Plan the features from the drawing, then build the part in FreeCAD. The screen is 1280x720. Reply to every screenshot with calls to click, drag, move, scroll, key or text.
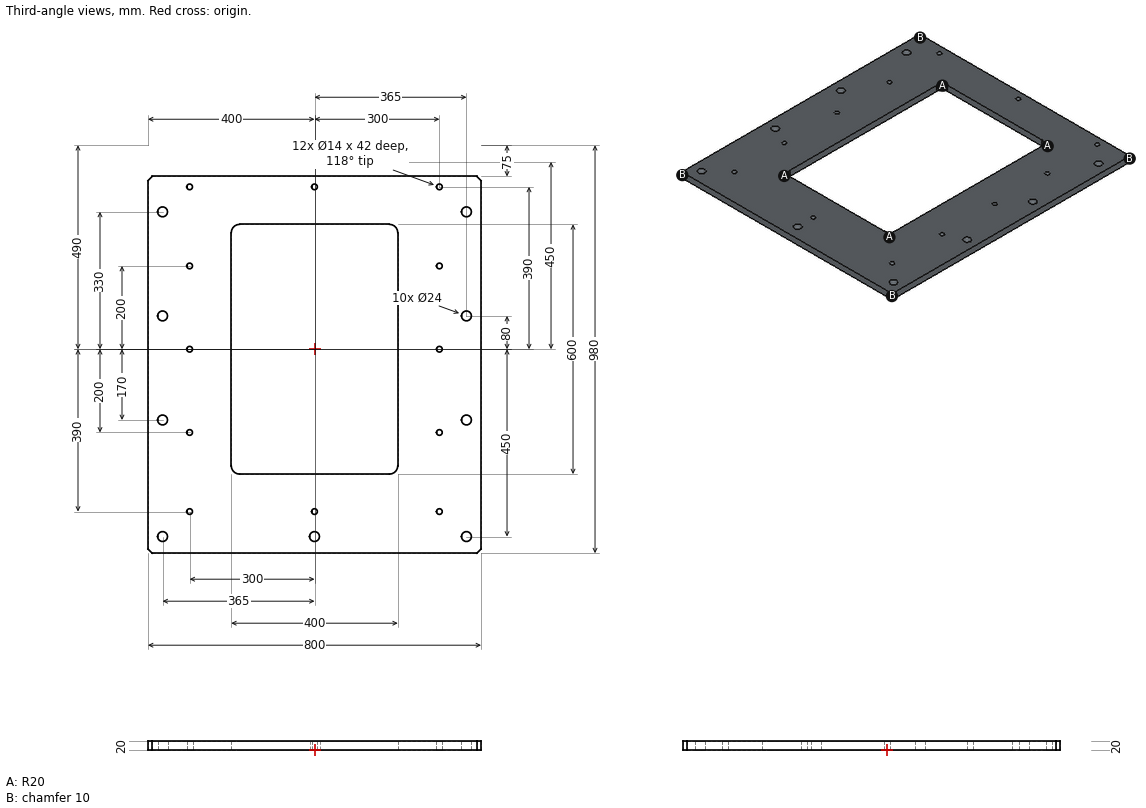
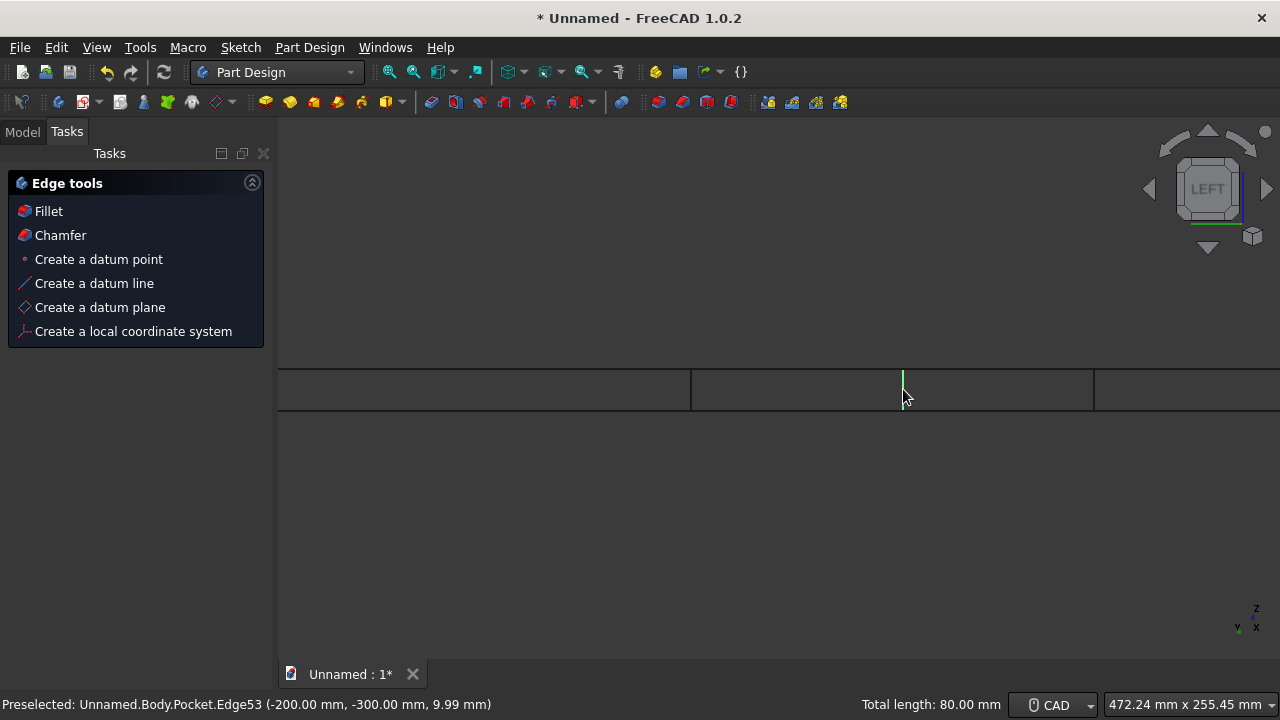
key(v)
key(1)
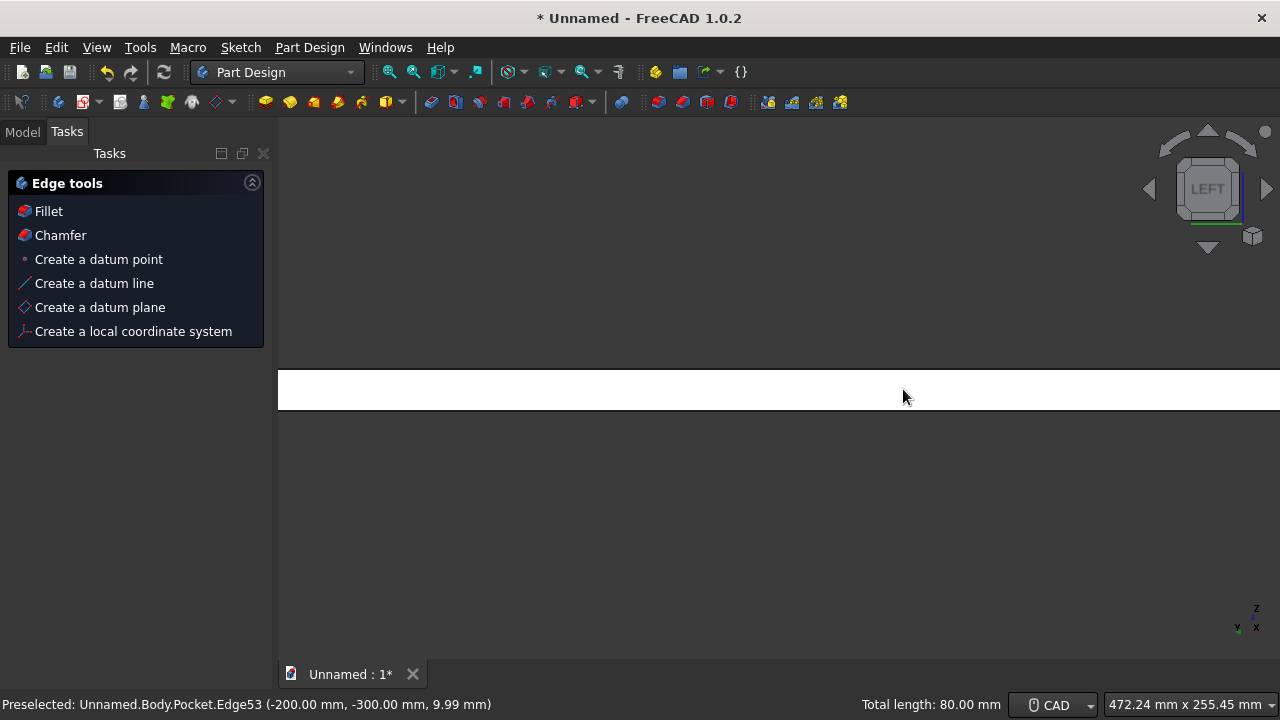
click(660, 102)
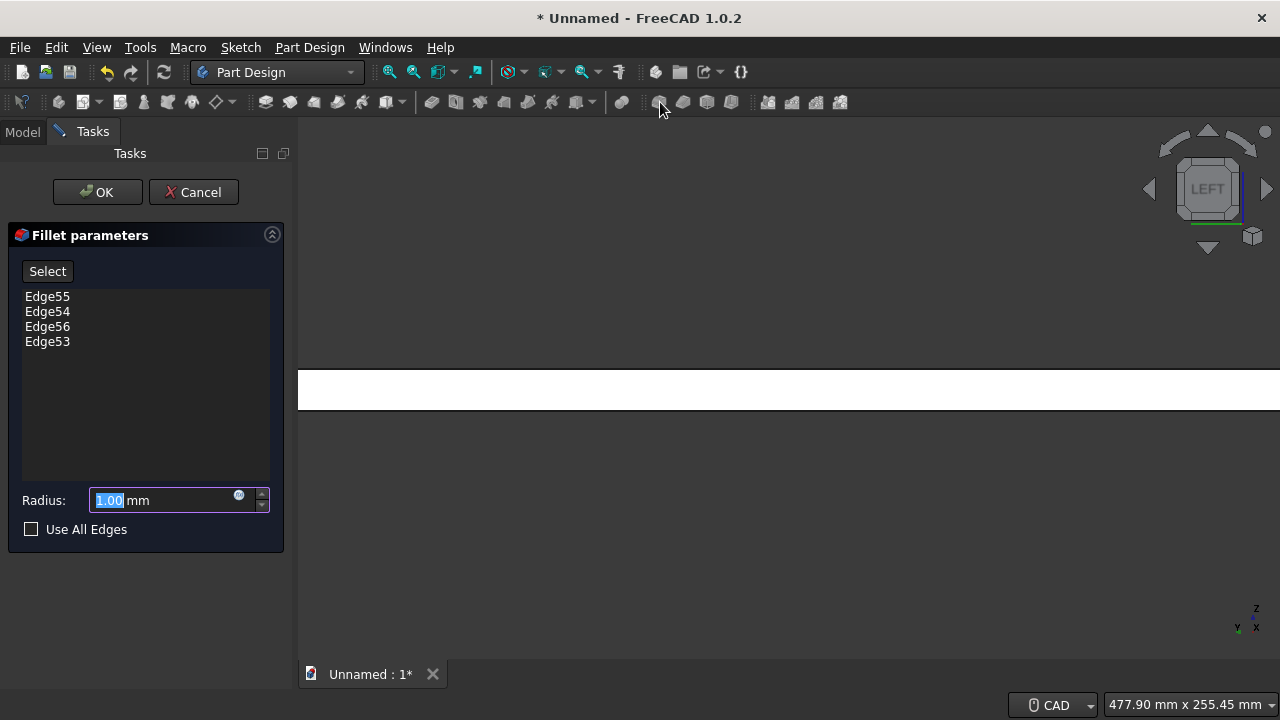
text(20)
key(Tab)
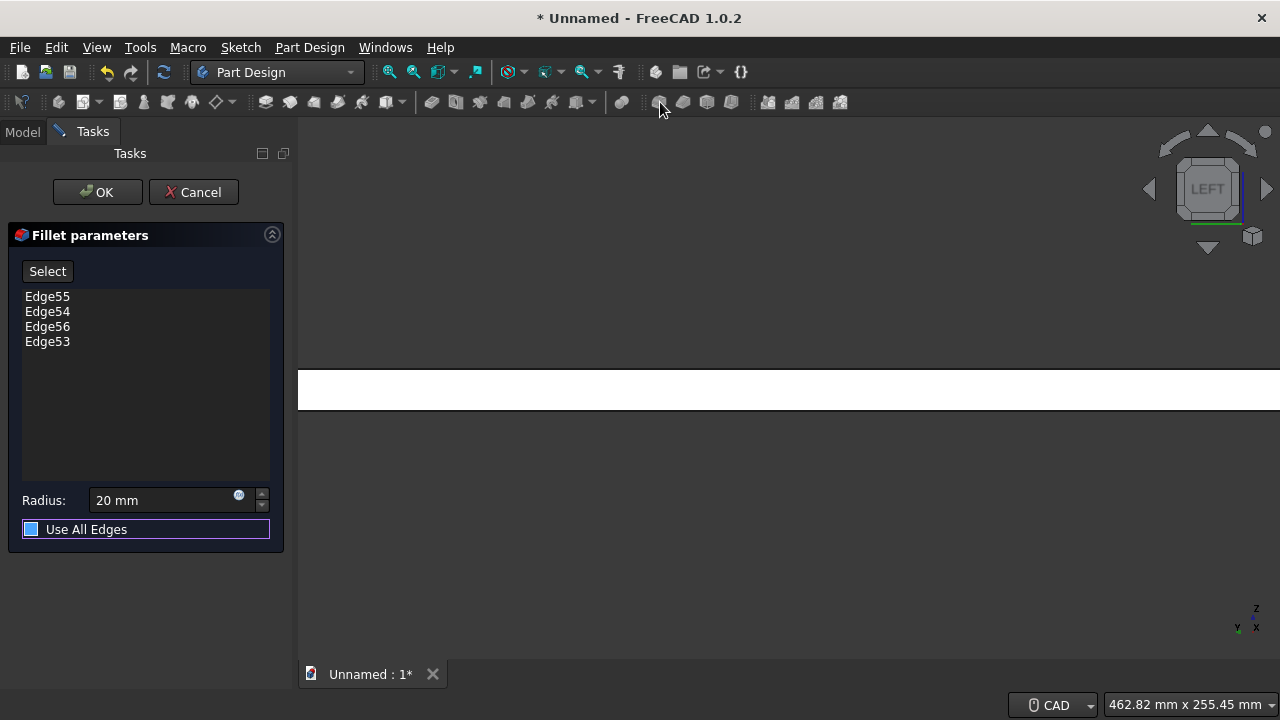
click(98, 192)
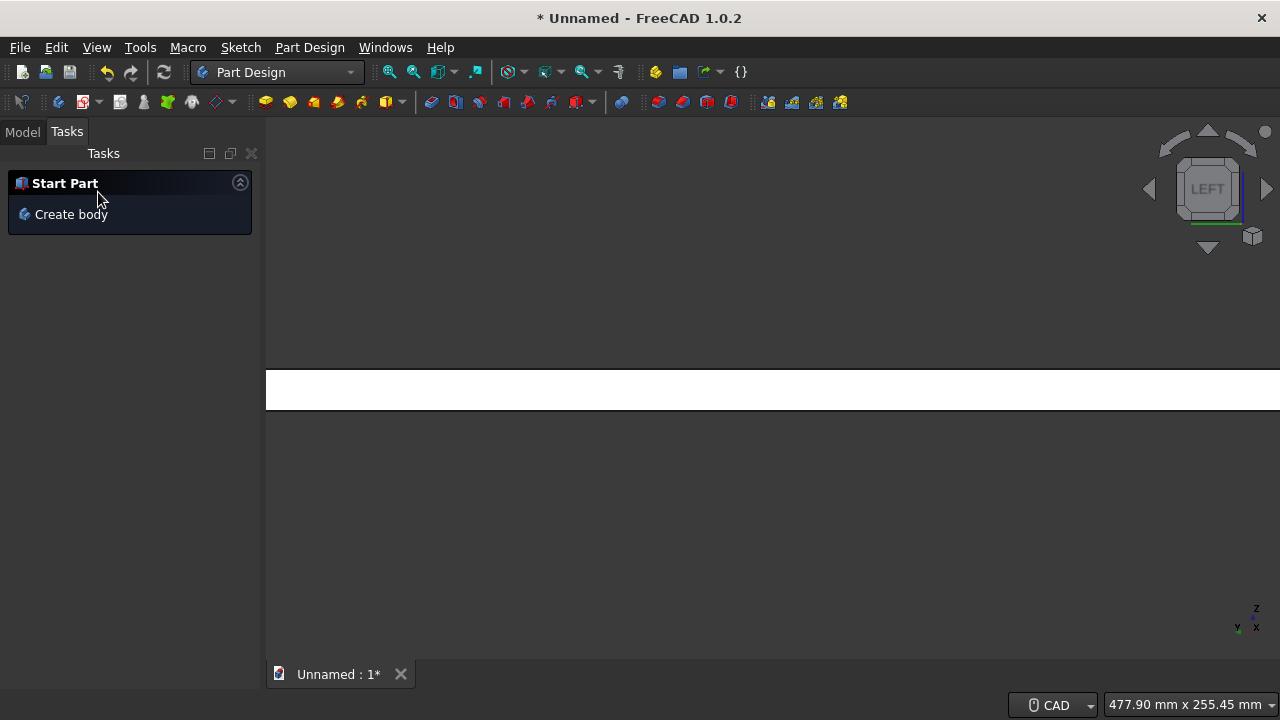
click(390, 72)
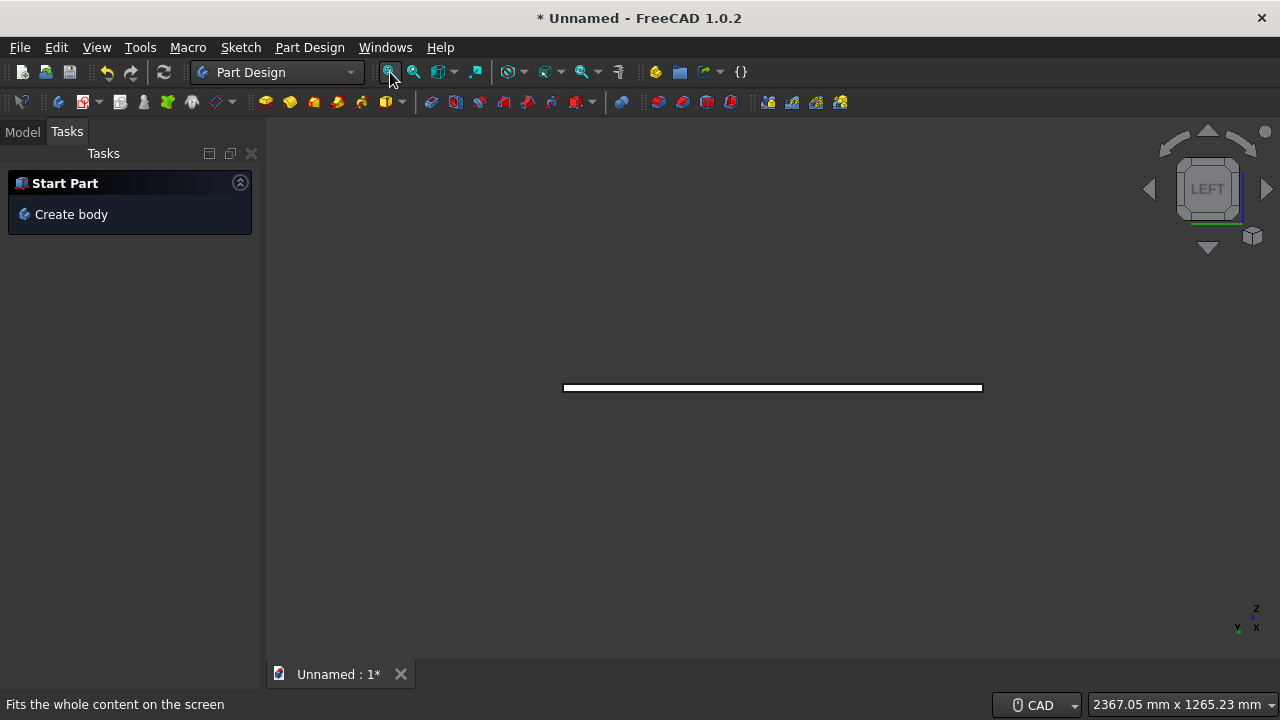
key(0)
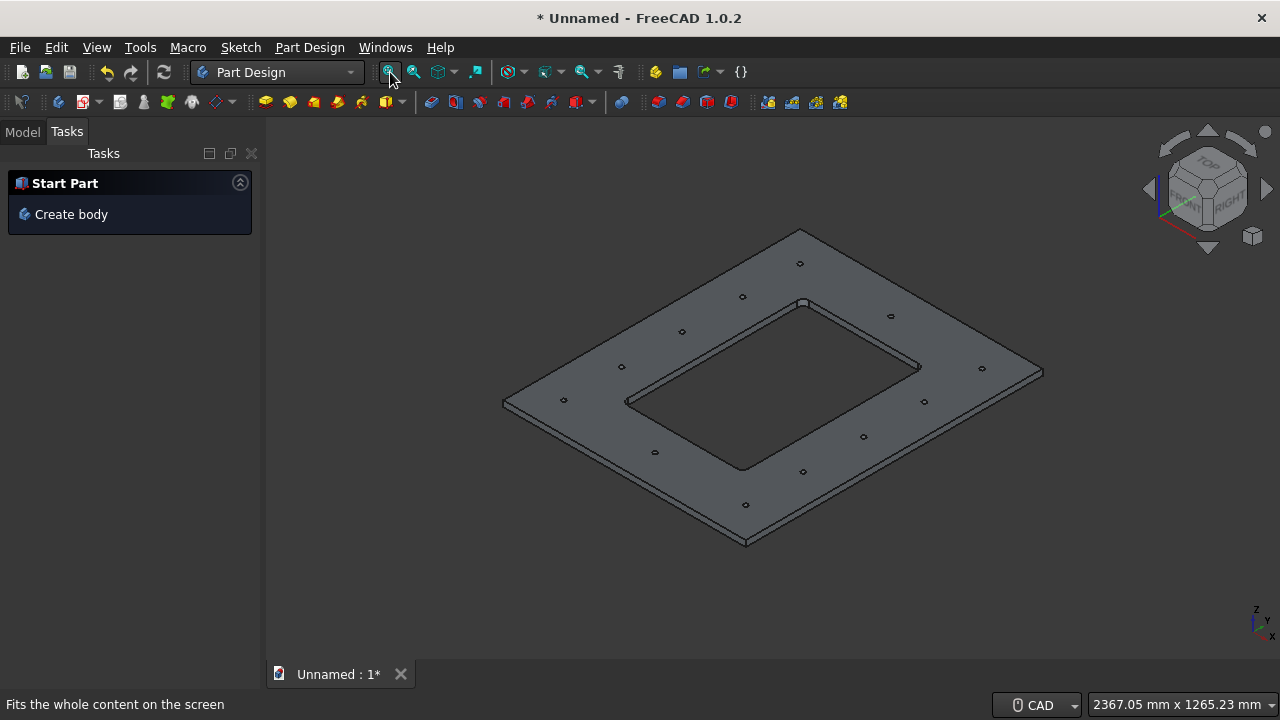
click(969, 350)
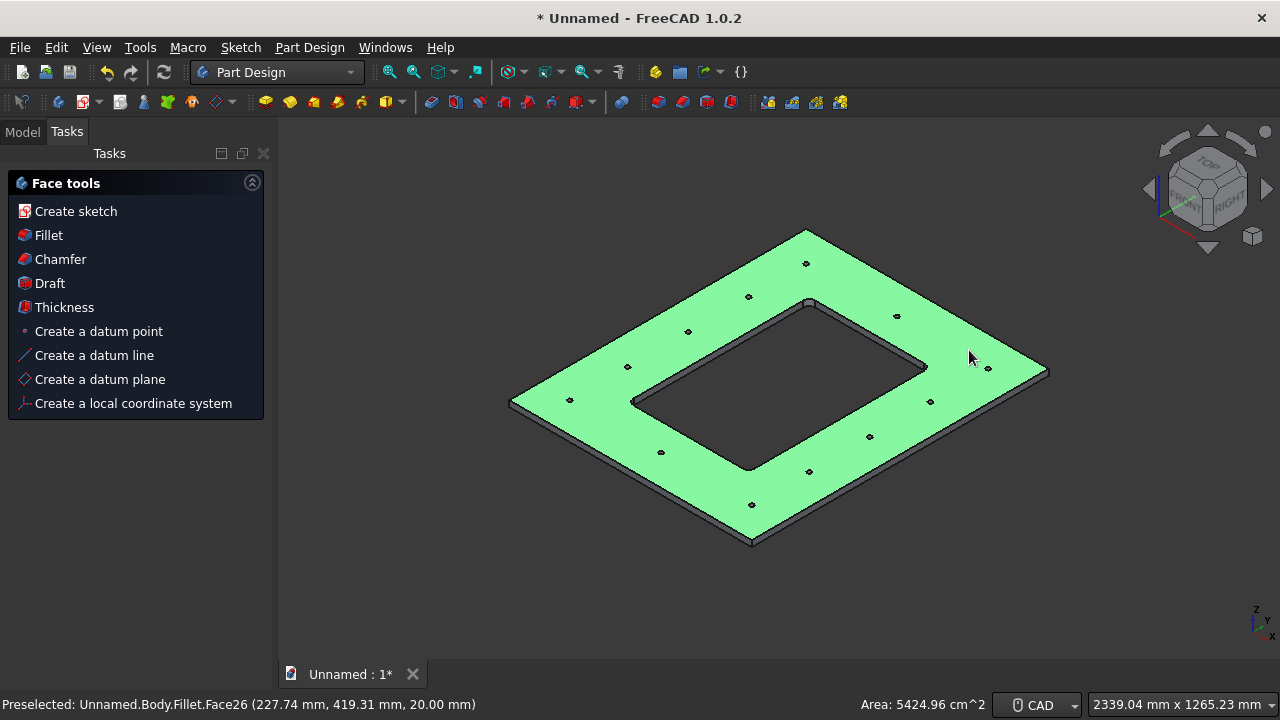
click(84, 102)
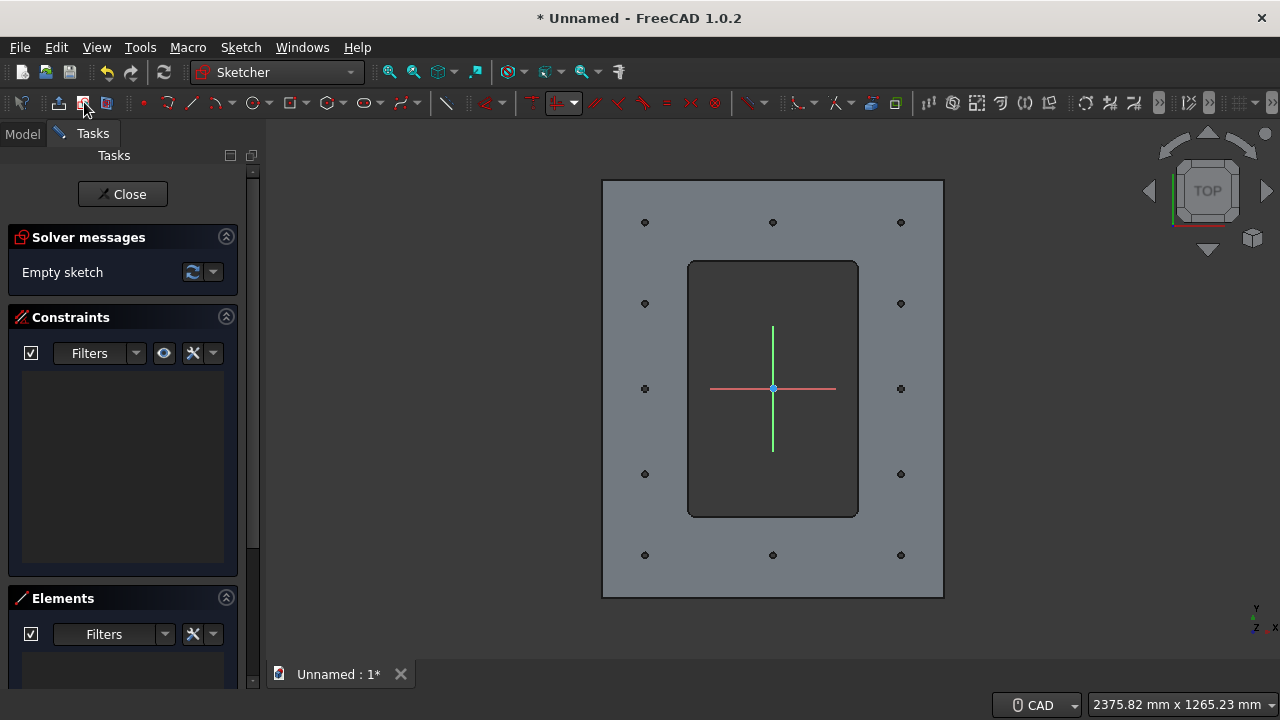
scroll(912, 147, up, 2)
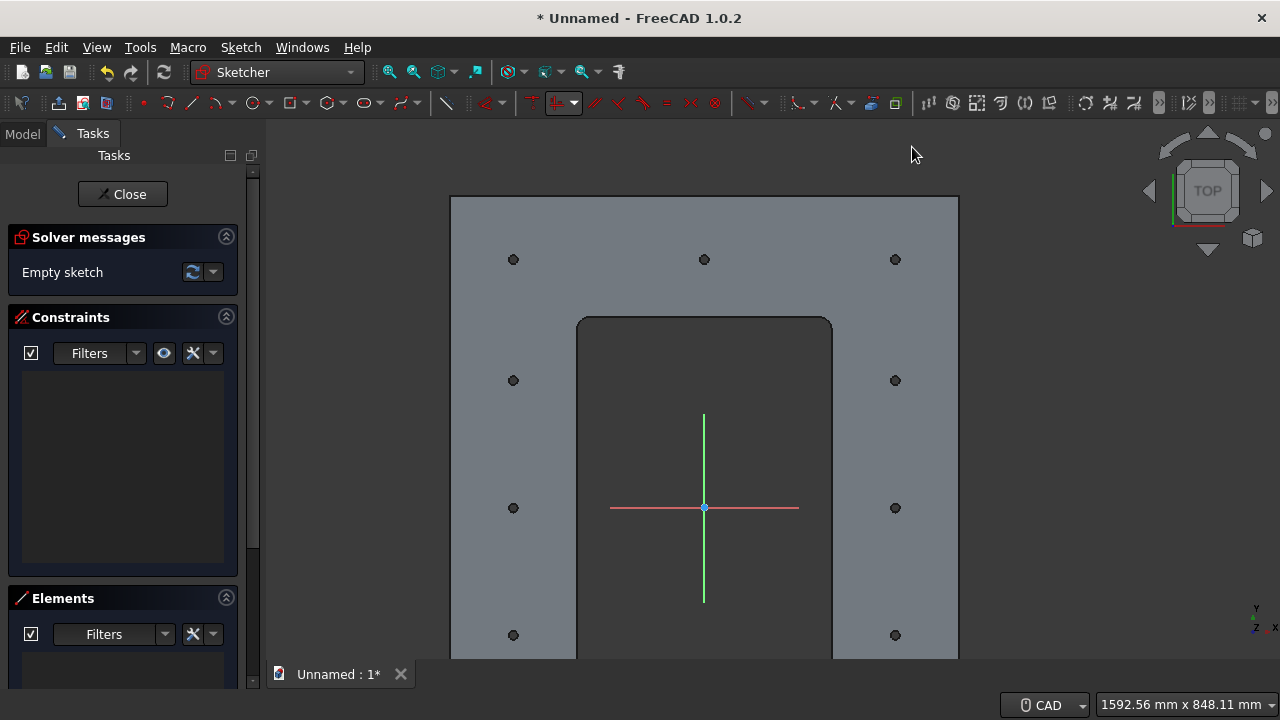
click(308, 104)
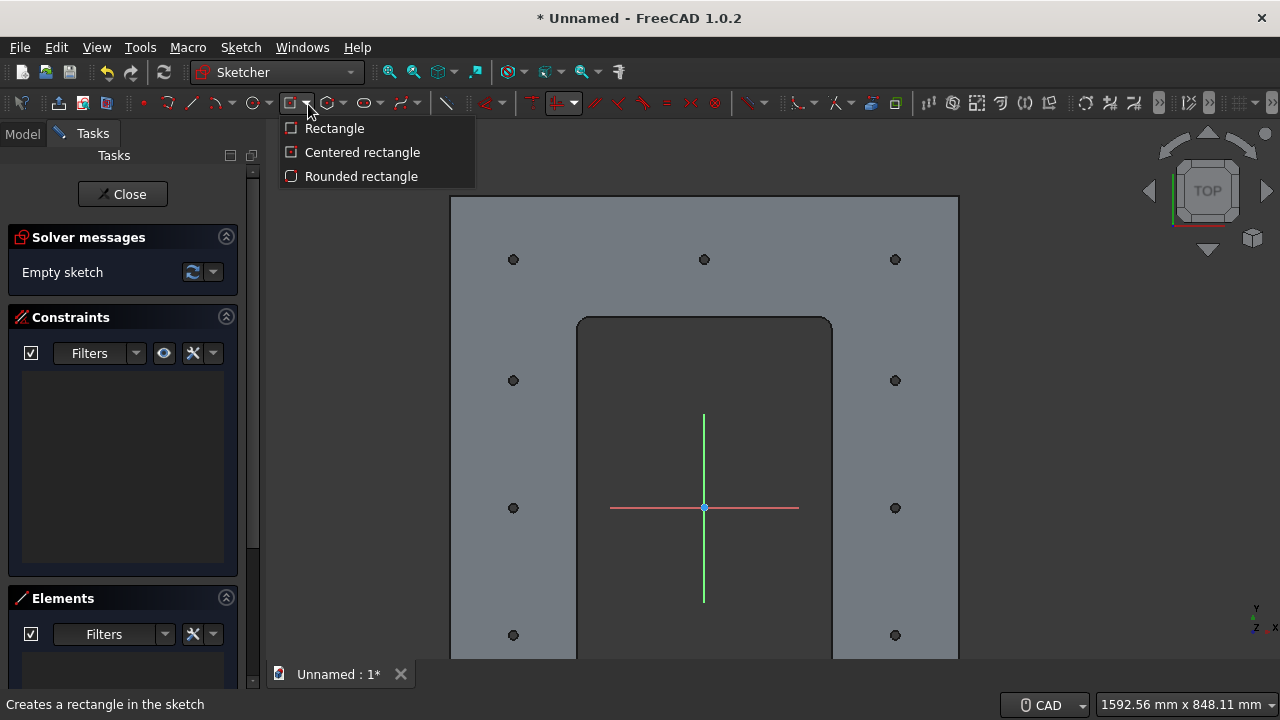
click(378, 128)